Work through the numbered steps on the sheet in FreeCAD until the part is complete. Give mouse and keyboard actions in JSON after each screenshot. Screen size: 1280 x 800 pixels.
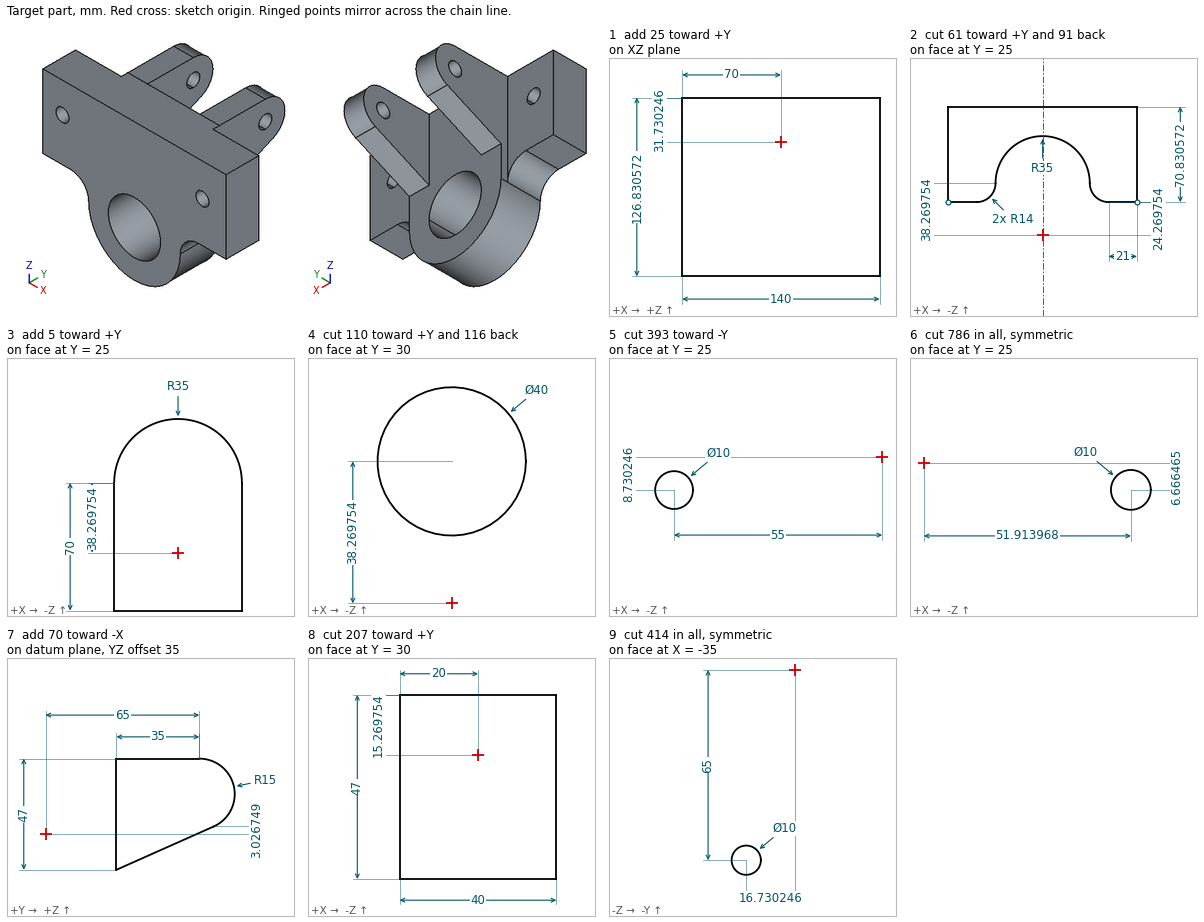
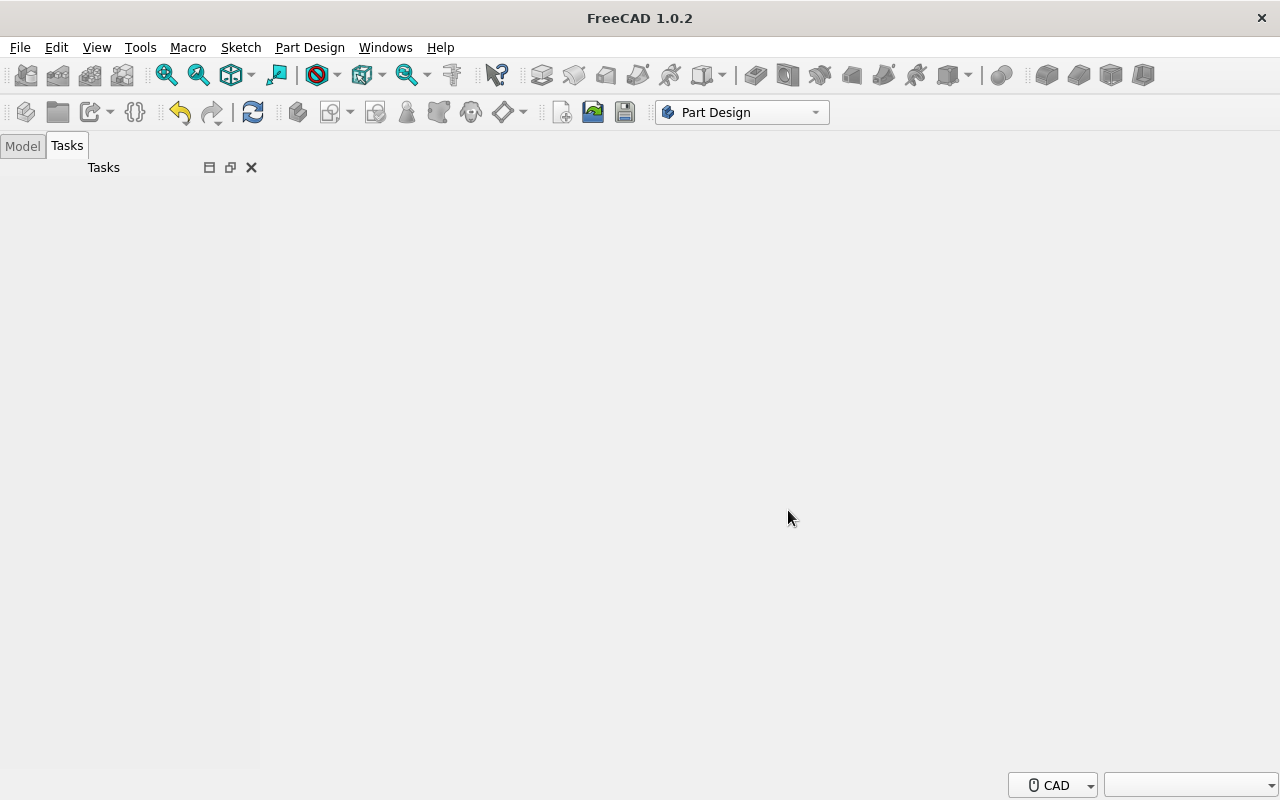
{"action": "left_click", "coordinate": [562, 112]}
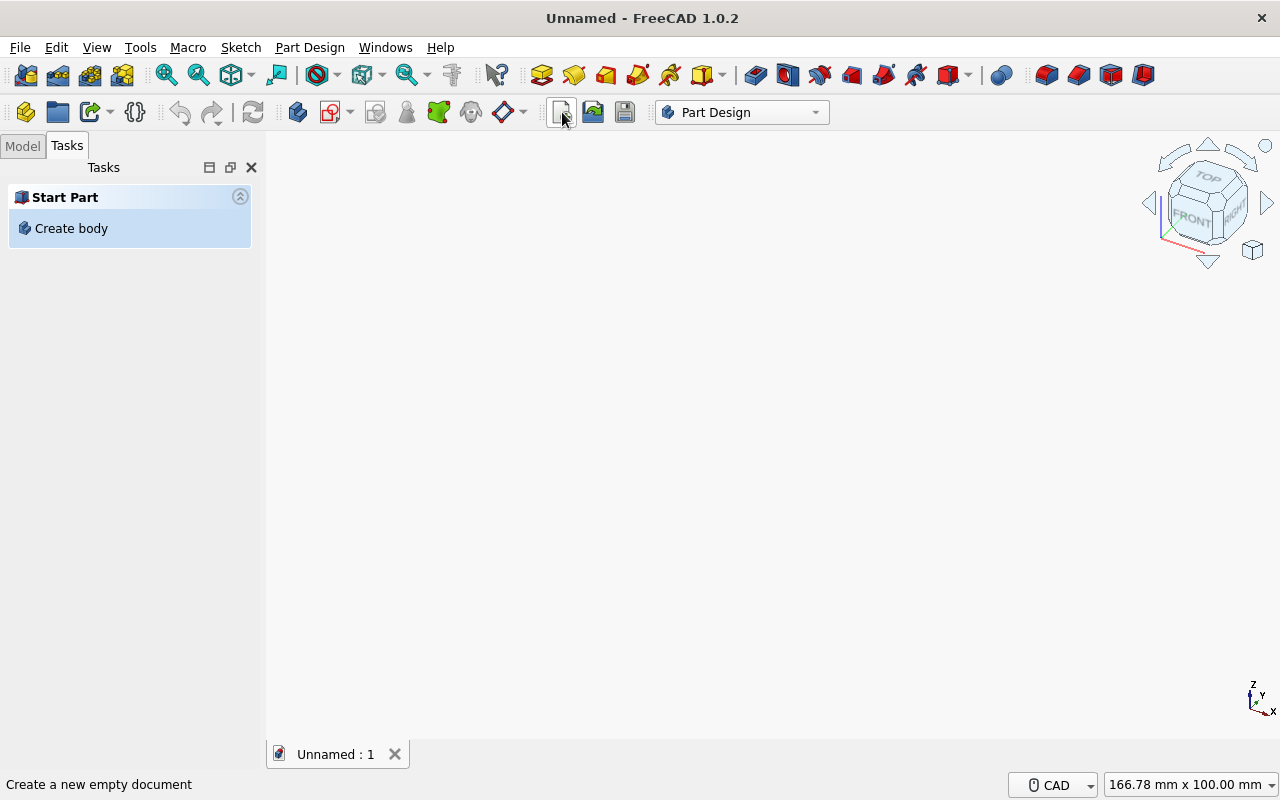
{"action": "left_click", "coordinate": [330, 112]}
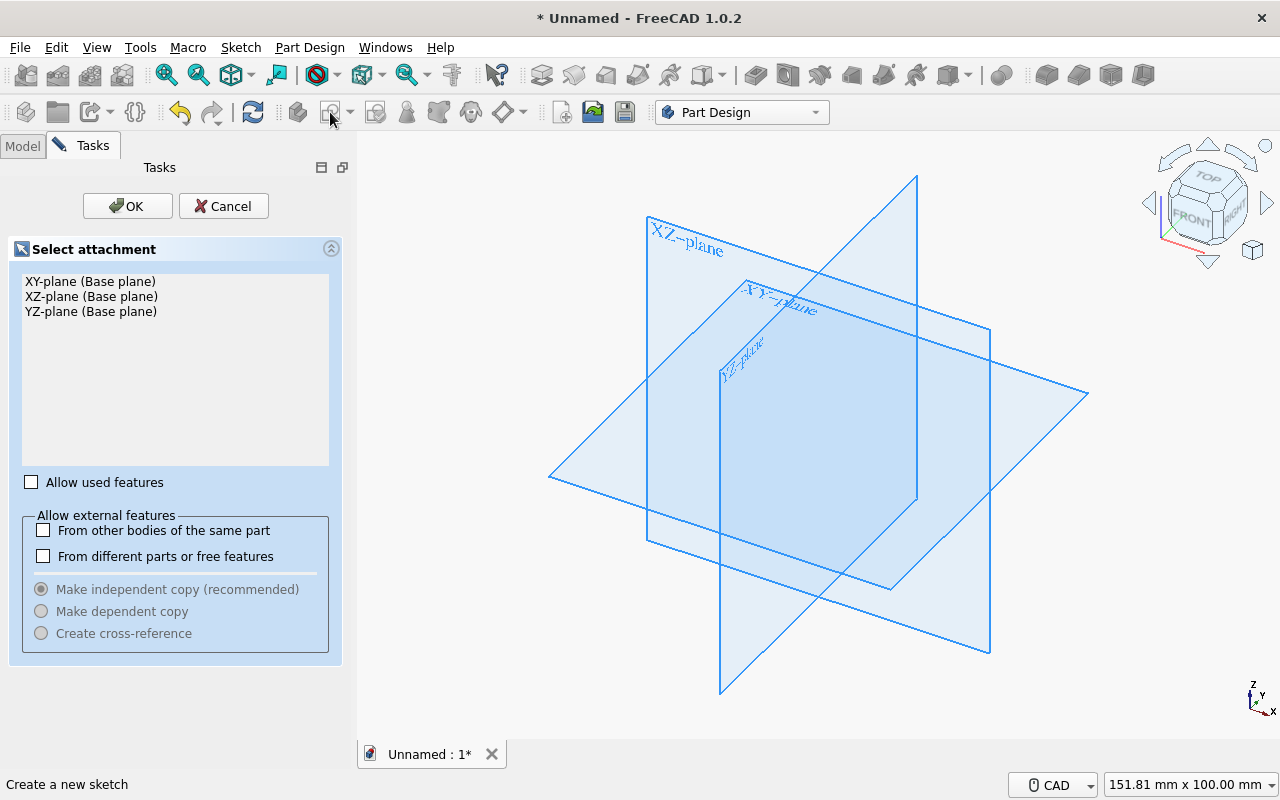
{"action": "left_click", "coordinate": [82, 296]}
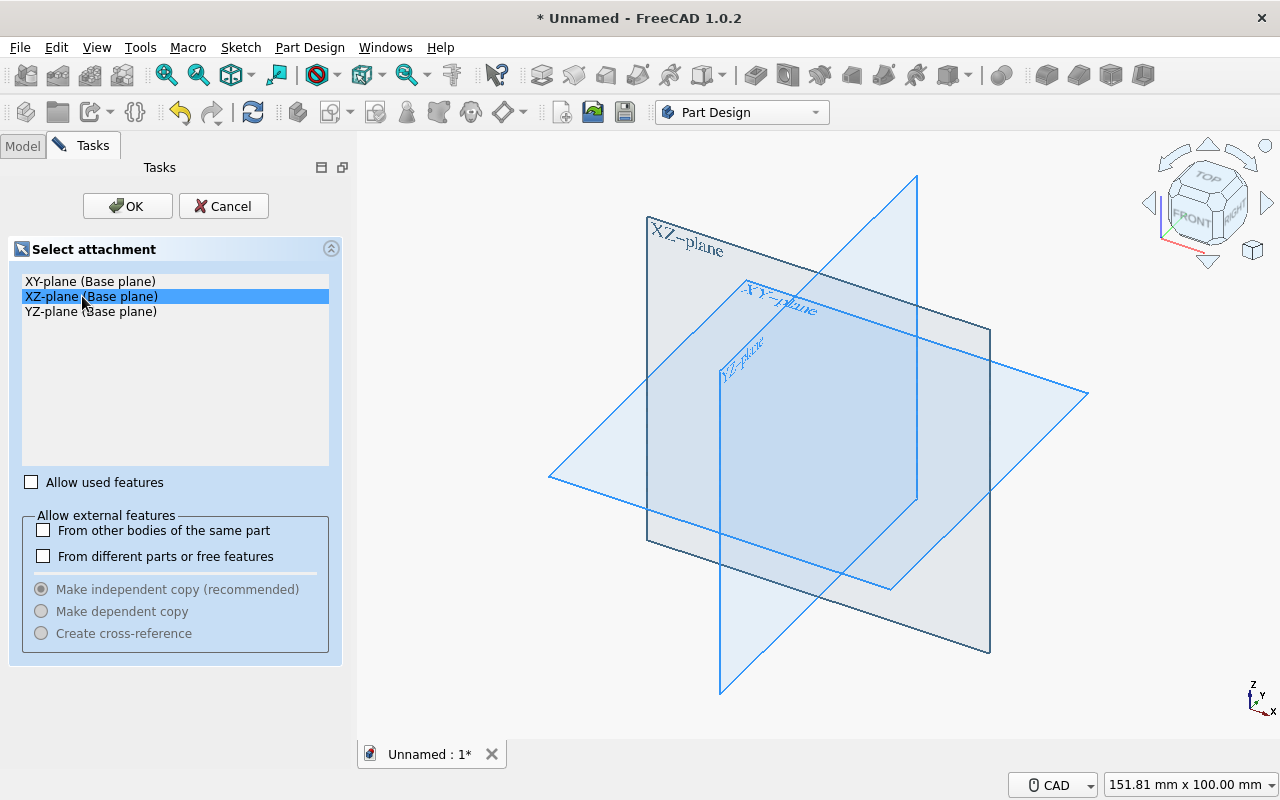
{"action": "left_click", "coordinate": [128, 206]}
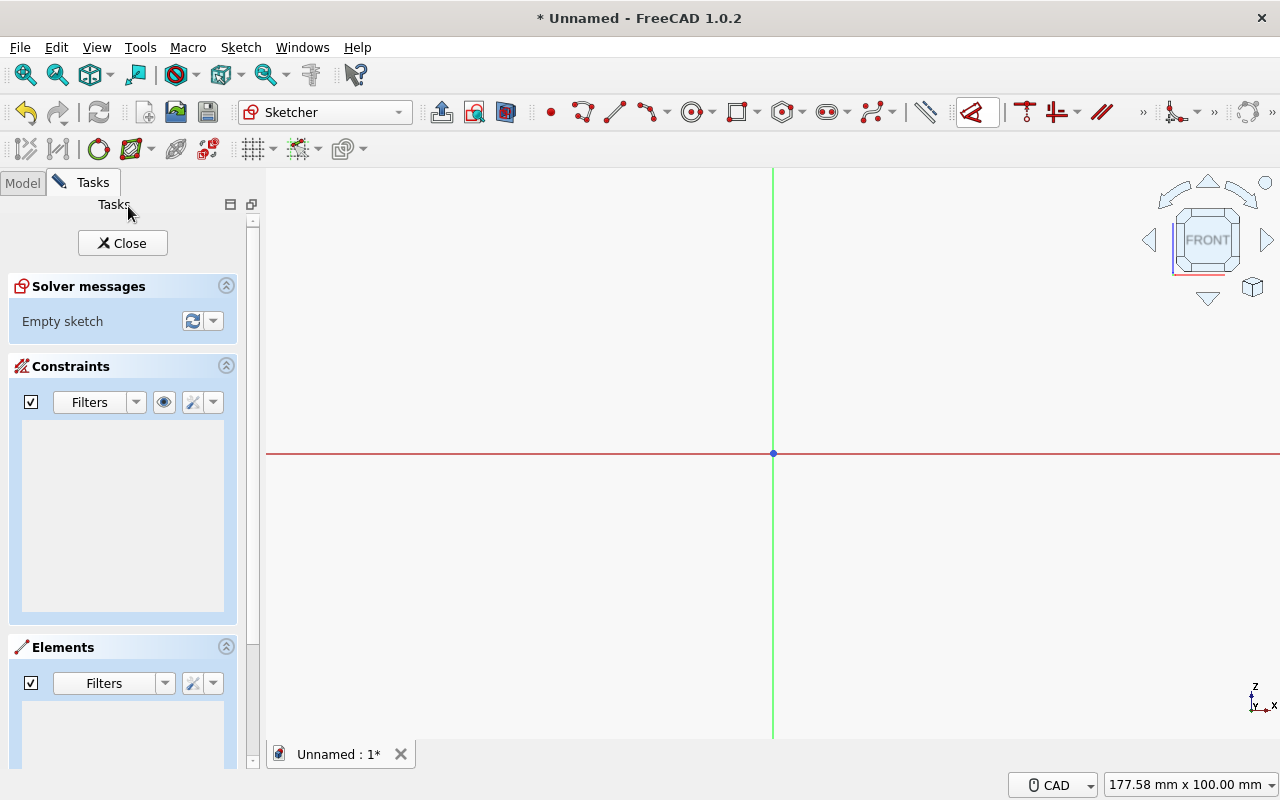
{"action": "scroll", "coordinate": [621, 233], "scroll_direction": "down", "scroll_amount": 3}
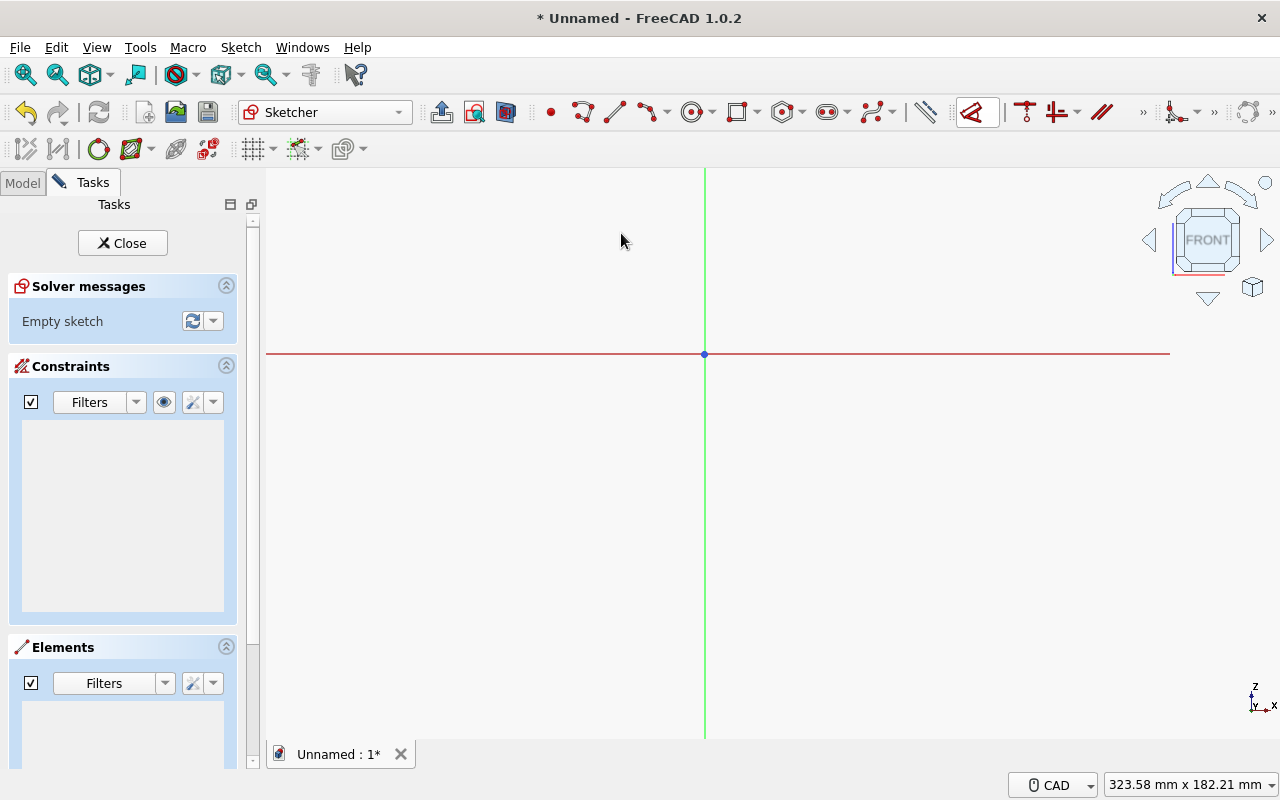
{"action": "left_click", "coordinate": [738, 112]}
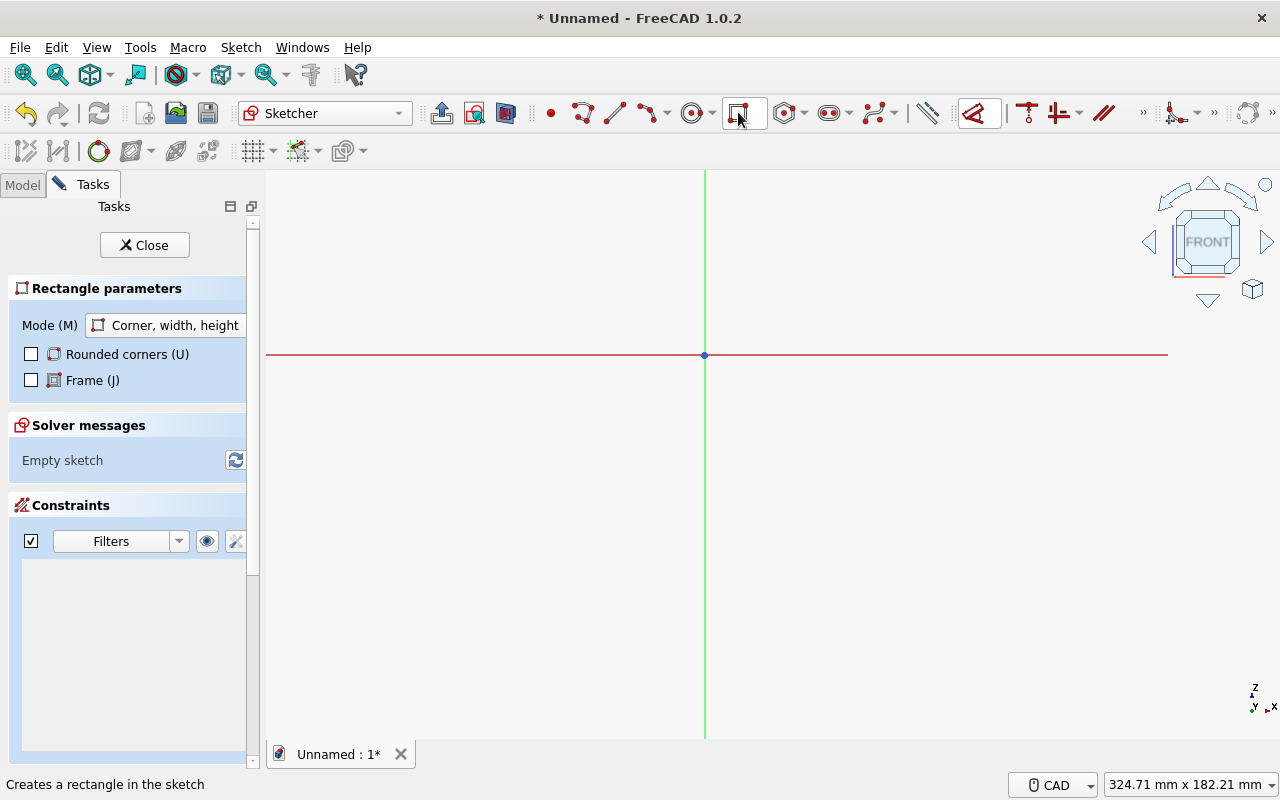
{"action": "left_click", "coordinate": [486, 256]}
{"action": "left_click", "coordinate": [923, 652]}
{"action": "key", "text": "Escape"}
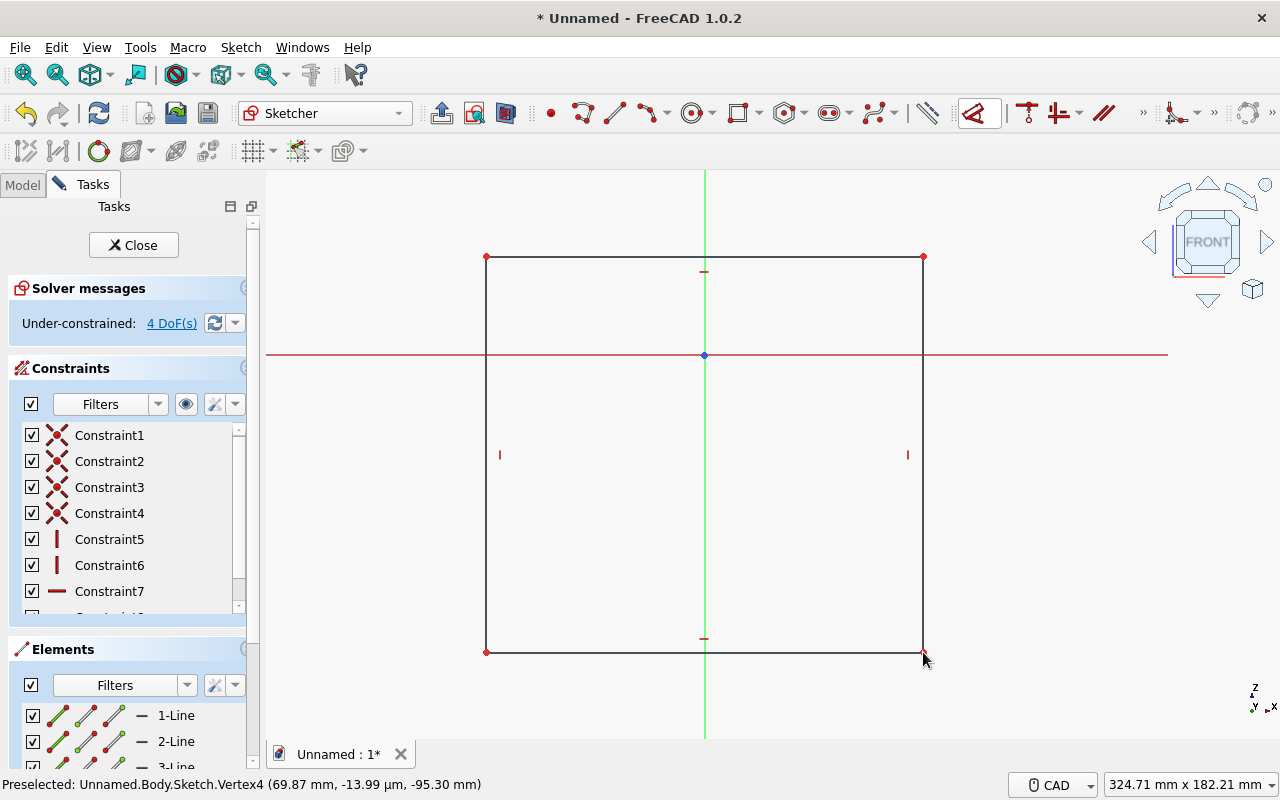
{"action": "left_click", "coordinate": [617, 653]}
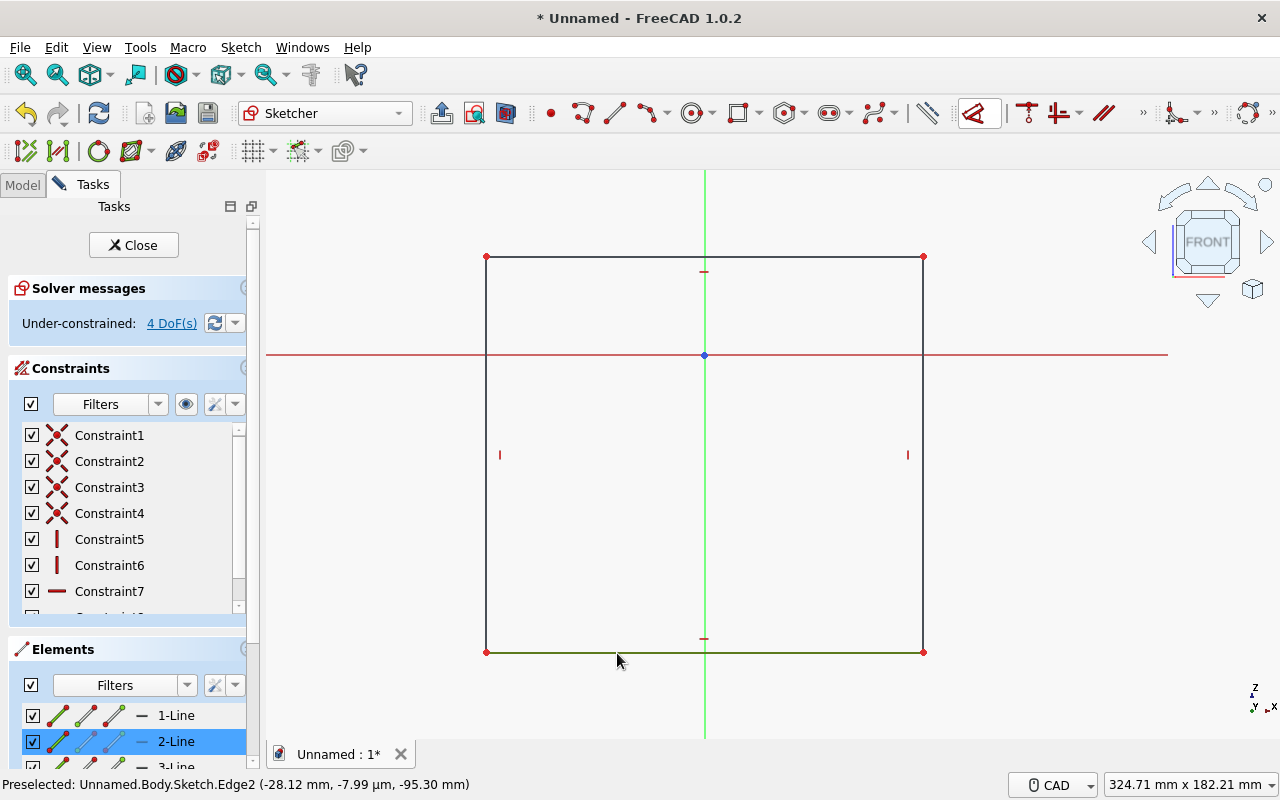
{"action": "key", "text": "l"}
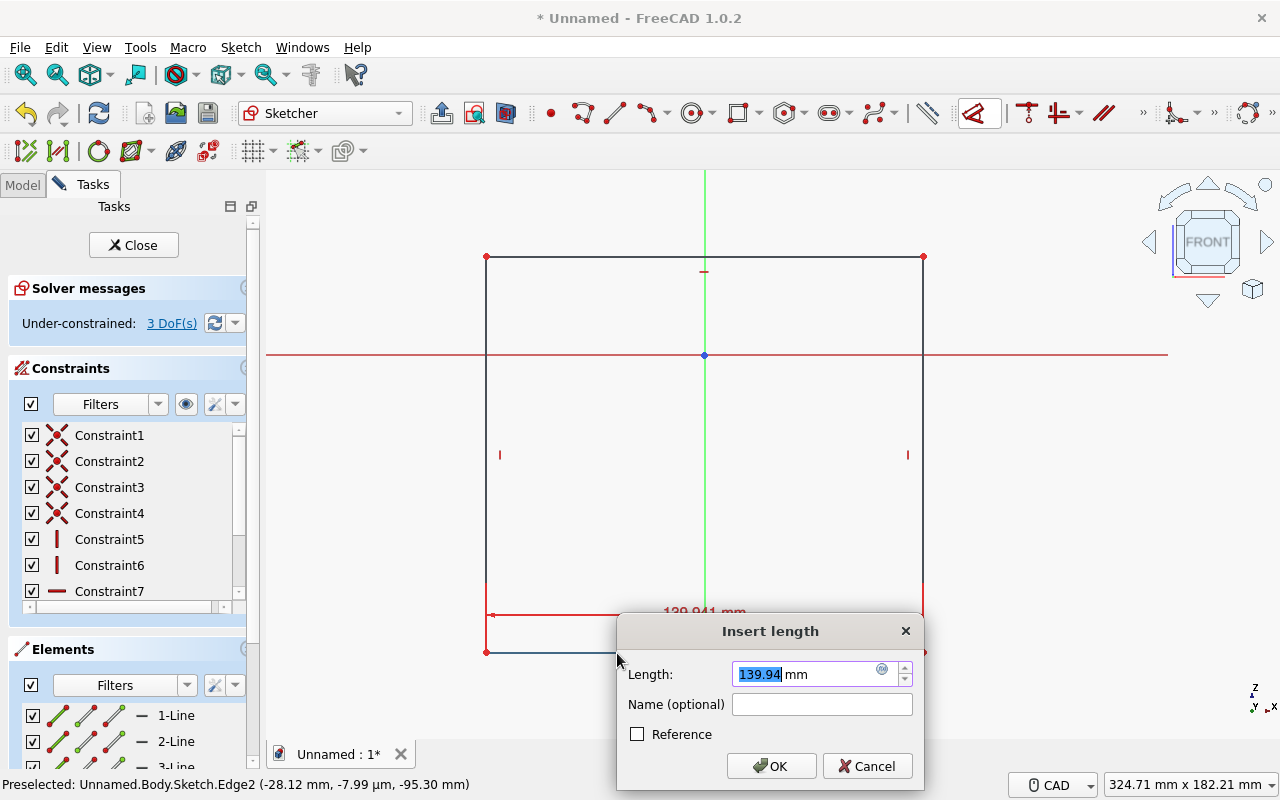
{"action": "type", "text": "140"}
{"action": "key", "text": "Return"}